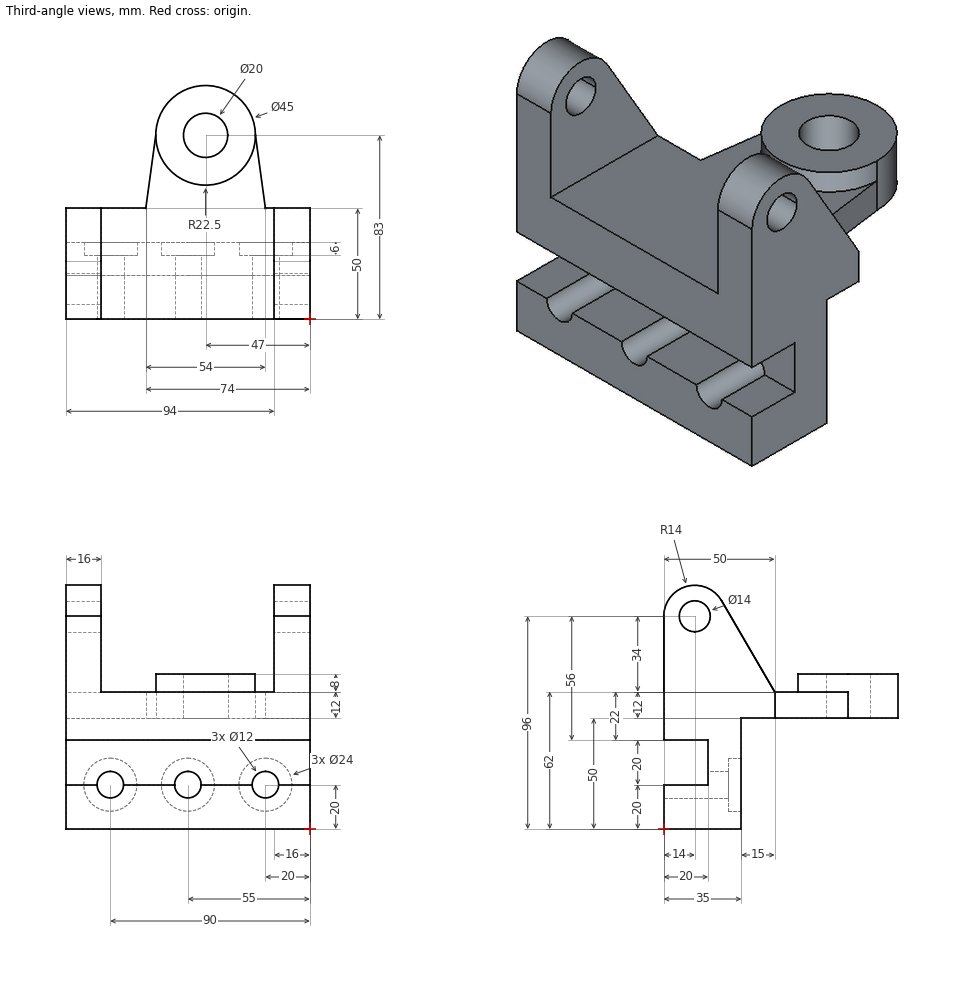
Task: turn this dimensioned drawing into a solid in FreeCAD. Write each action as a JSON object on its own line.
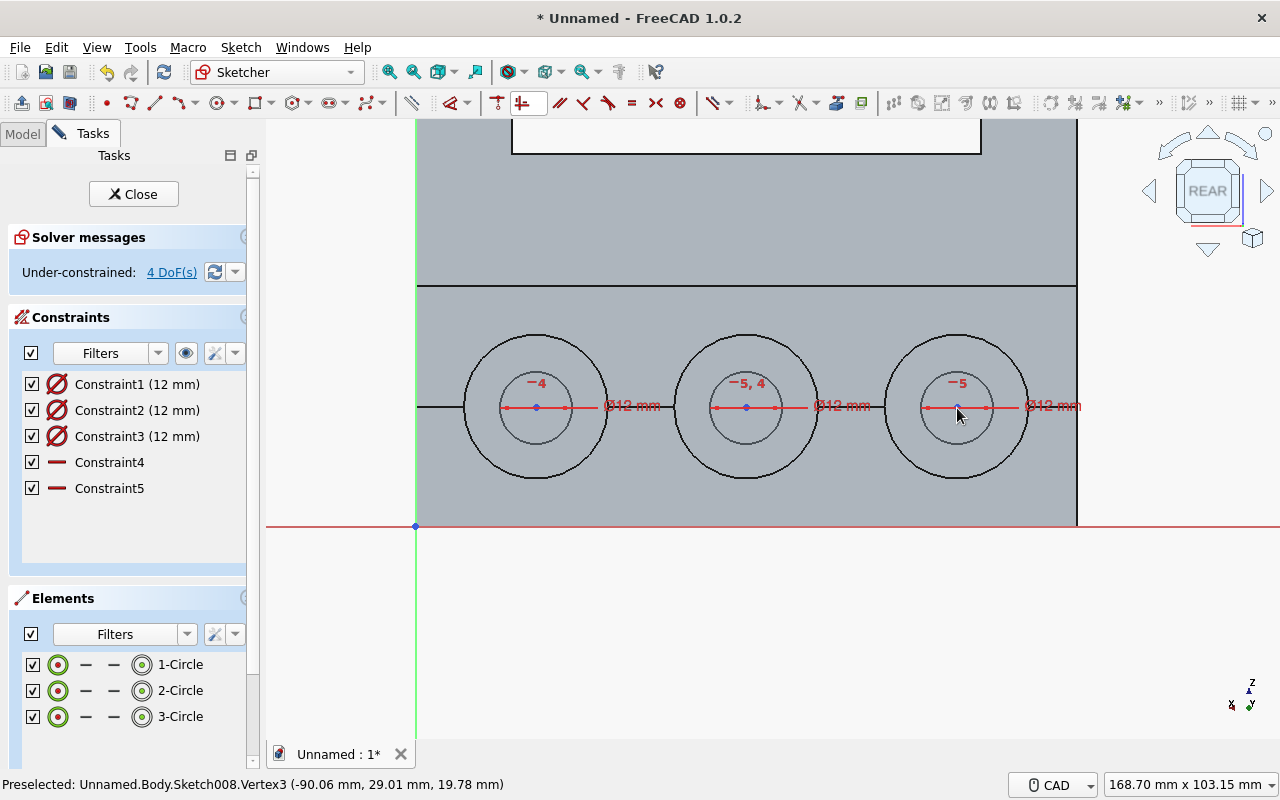
{"action": "left_click", "coordinate": [450, 104]}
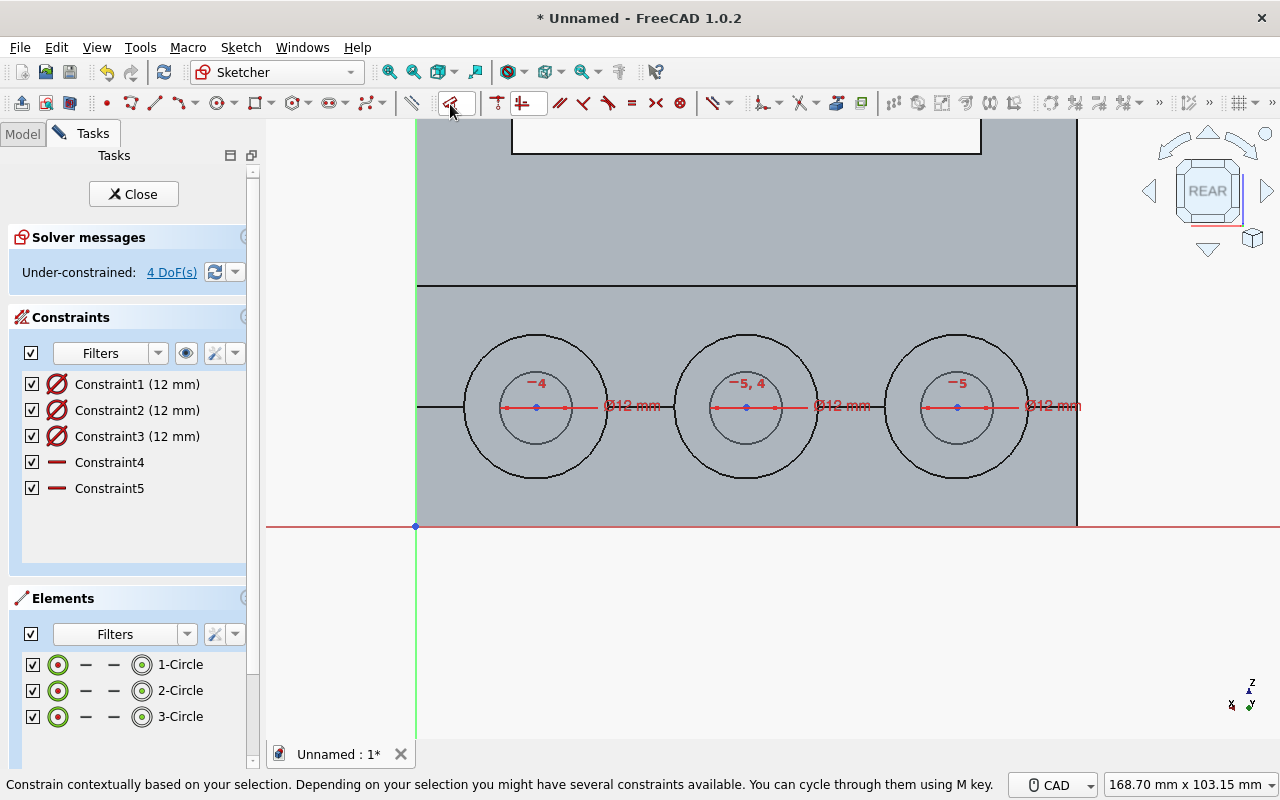
{"action": "left_click", "coordinate": [536, 408]}
{"action": "left_click", "coordinate": [476, 561]}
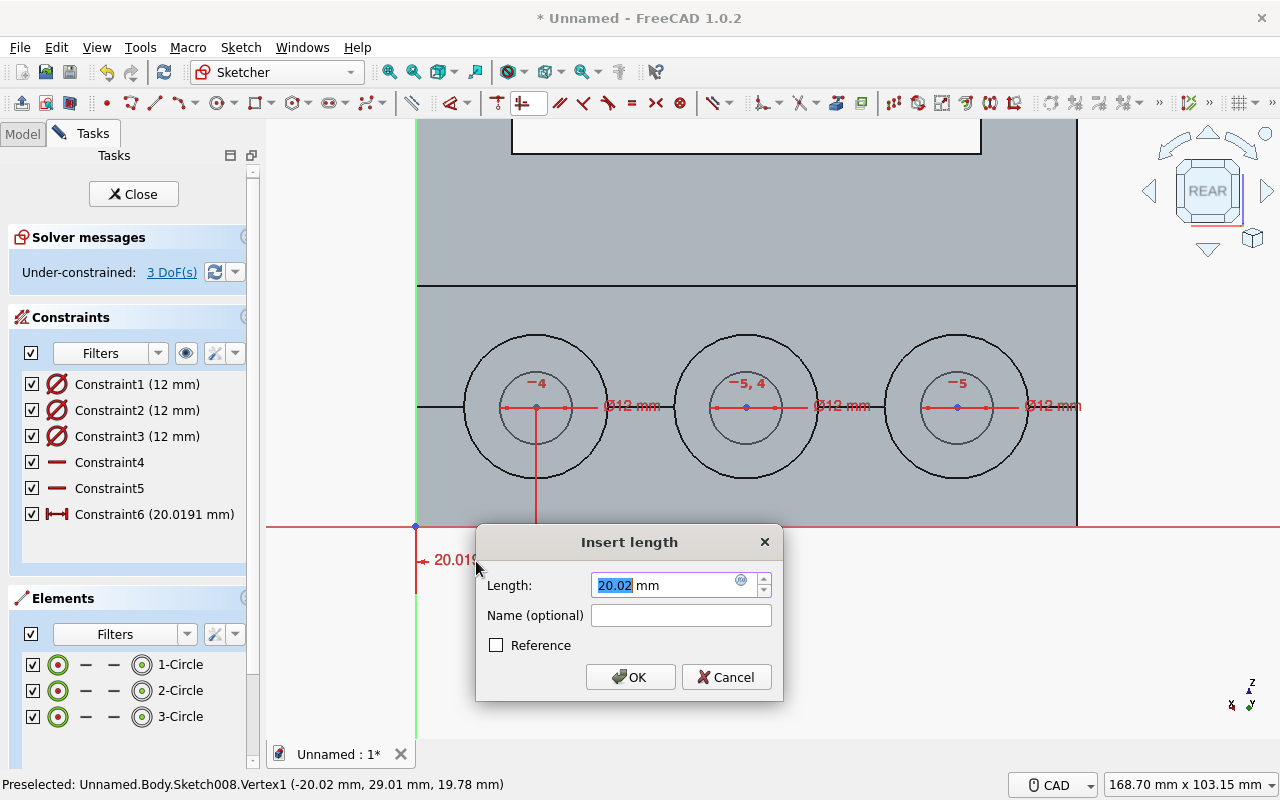
{"action": "type", "text": "20"}
{"action": "key", "text": "Return"}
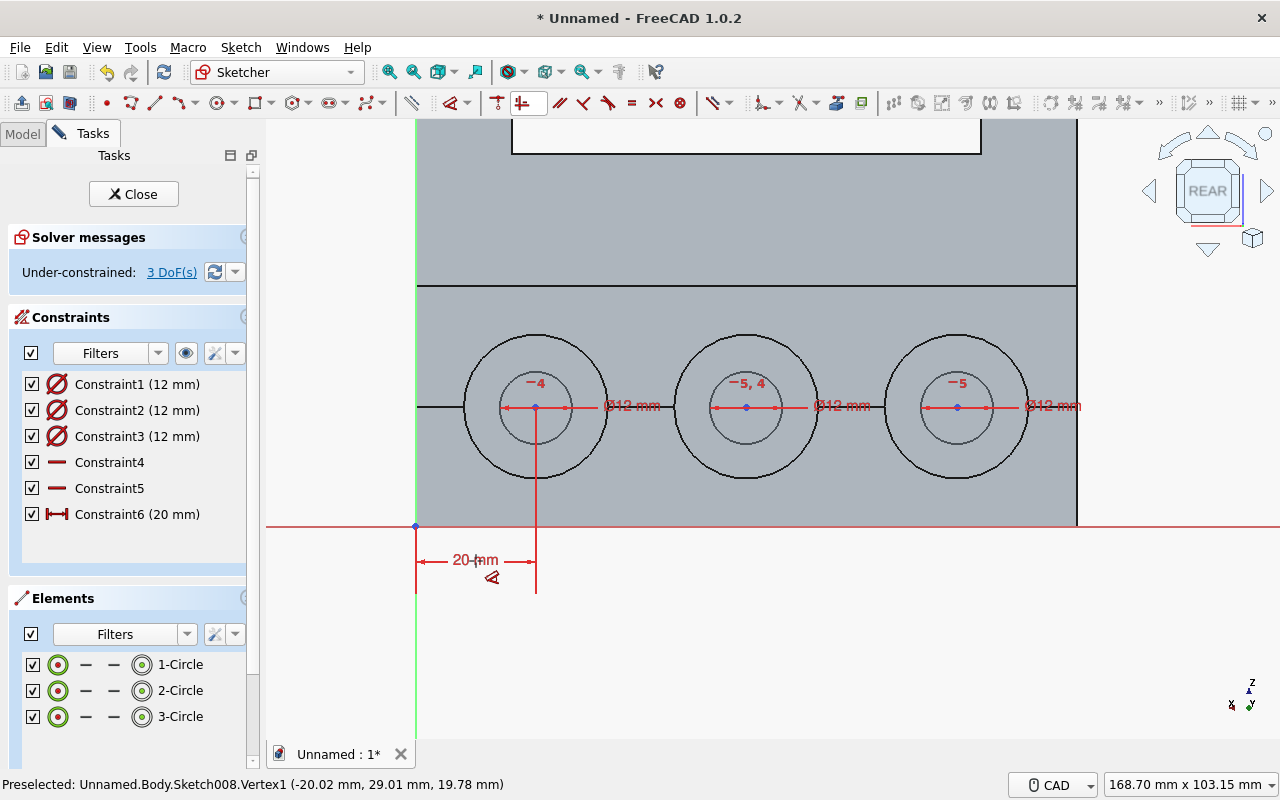
{"action": "left_click", "coordinate": [536, 408]}
{"action": "left_click", "coordinate": [382, 467]}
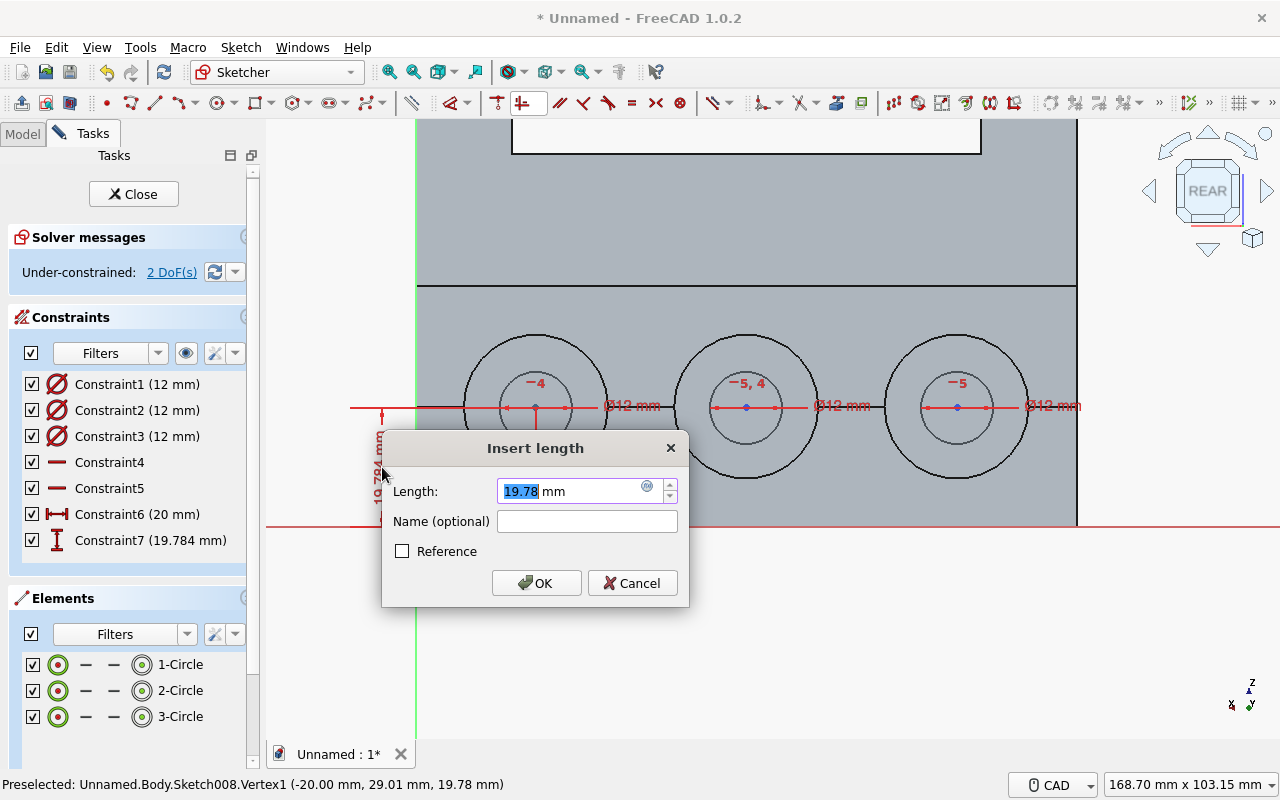
{"action": "type", "text": "20"}
{"action": "key", "text": "Return"}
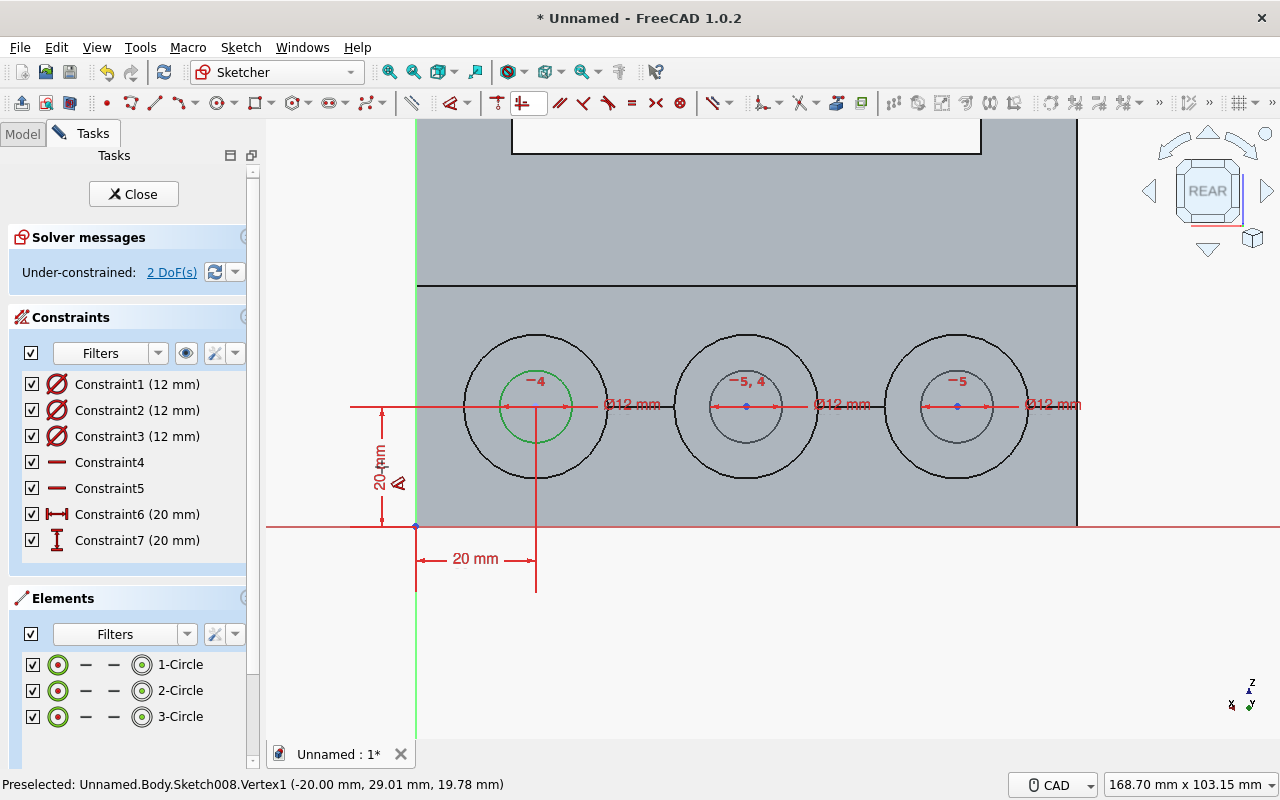
{"action": "left_click", "coordinate": [746, 407]}
{"action": "left_click", "coordinate": [581, 561]}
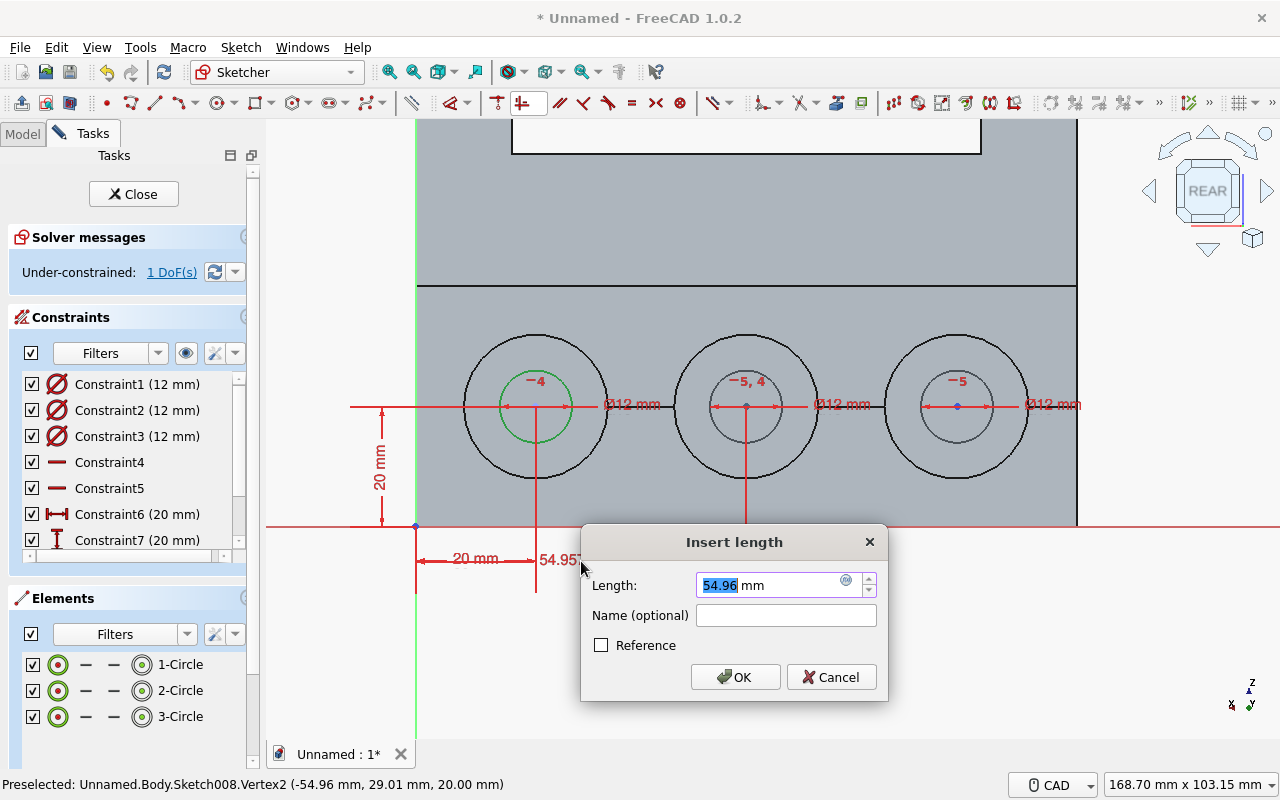
{"action": "type", "text": "55"}
{"action": "key", "text": "Return"}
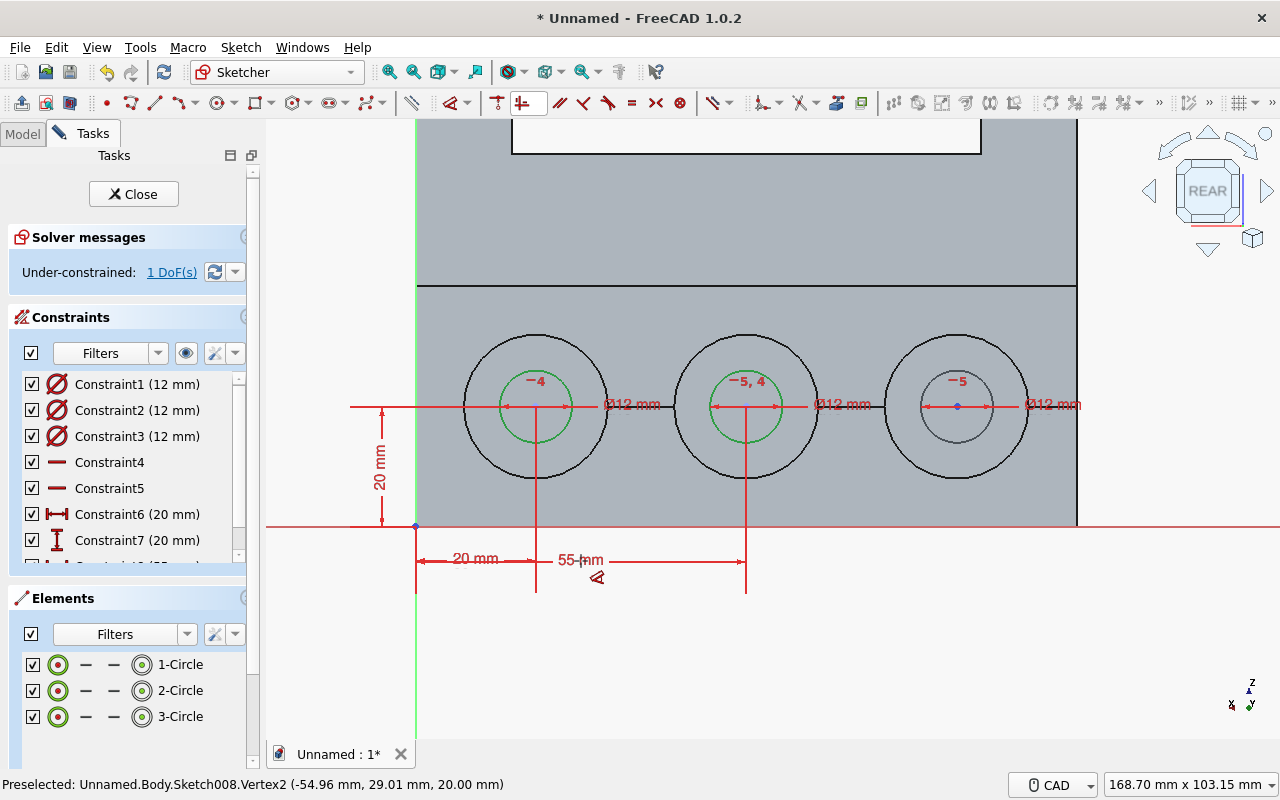
{"action": "left_click", "coordinate": [957, 407]}
{"action": "left_click", "coordinate": [686, 561]}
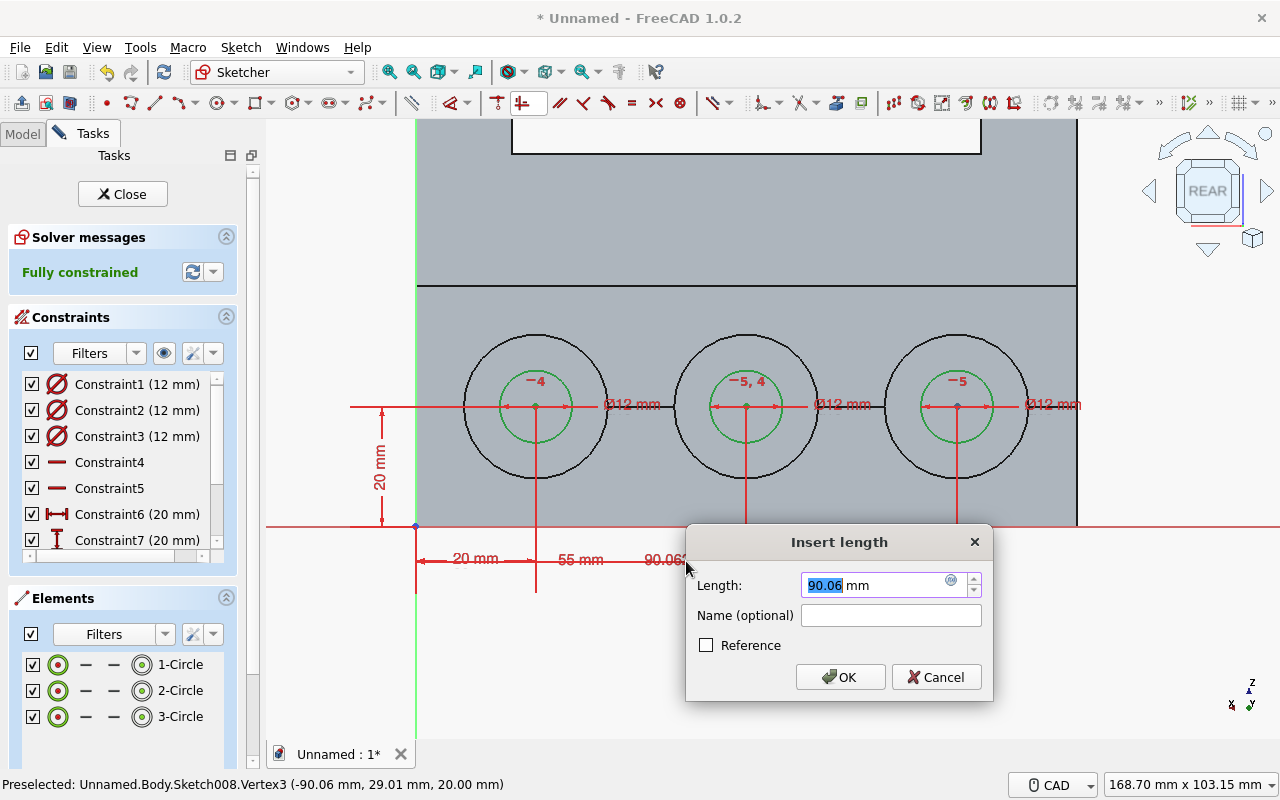
{"action": "type", "text": "90"}
{"action": "key", "text": "Return"}
{"action": "key", "text": "Escape"}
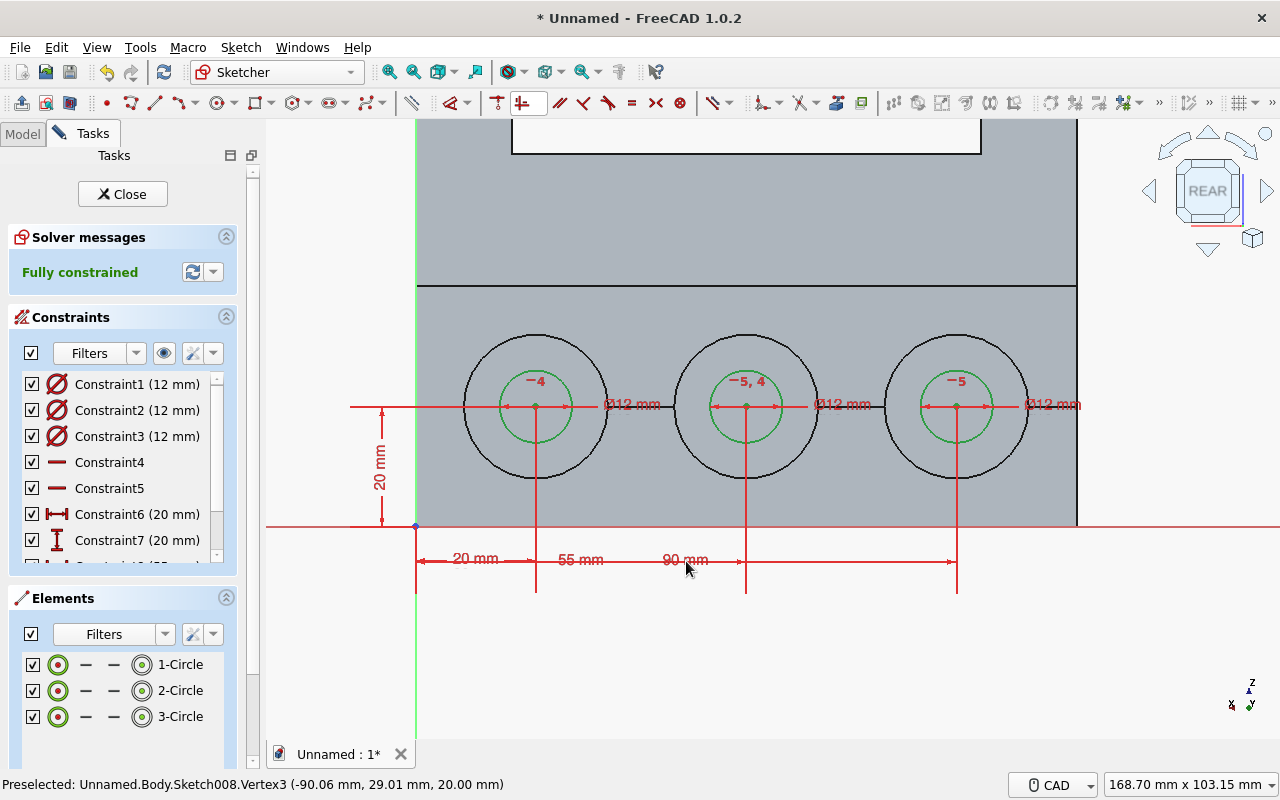
{"action": "left_click", "coordinate": [123, 194]}